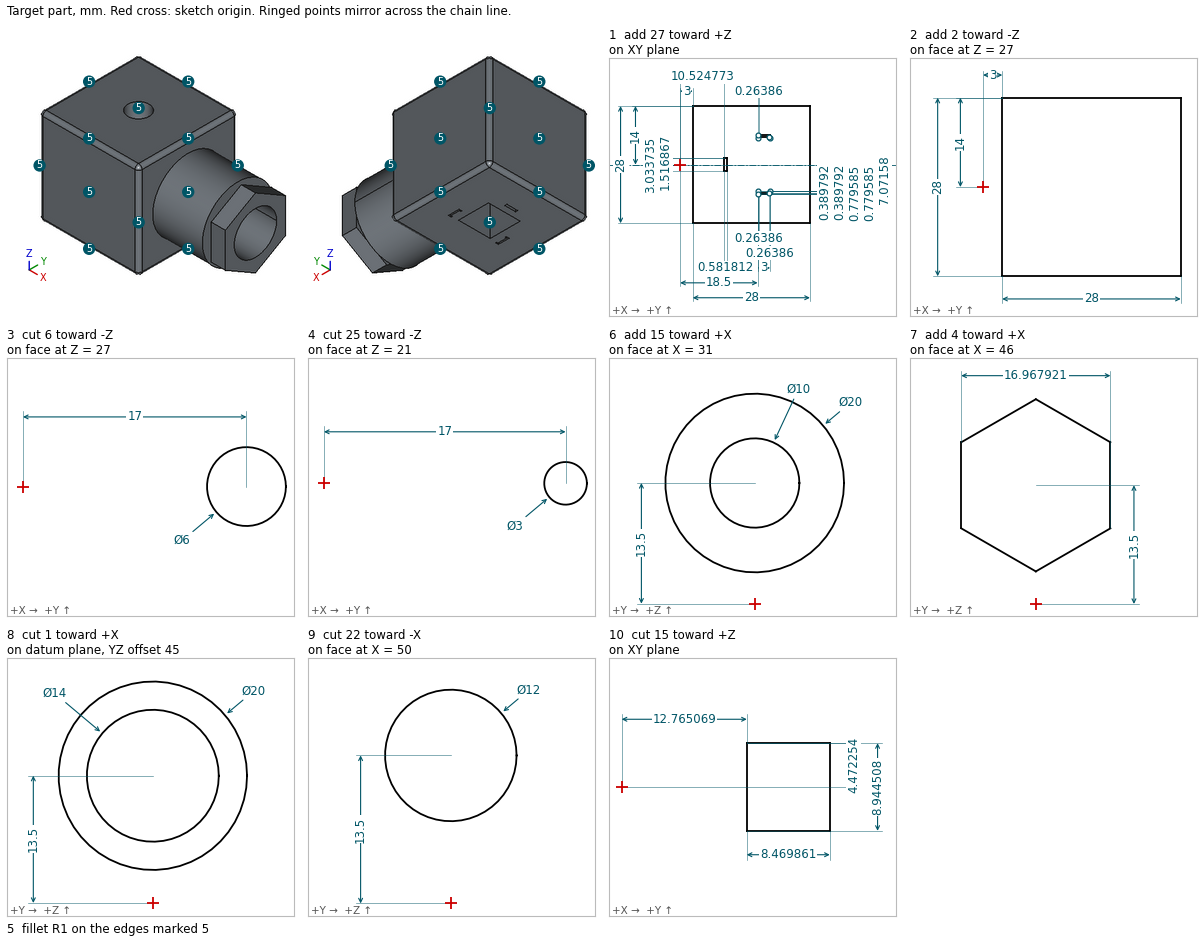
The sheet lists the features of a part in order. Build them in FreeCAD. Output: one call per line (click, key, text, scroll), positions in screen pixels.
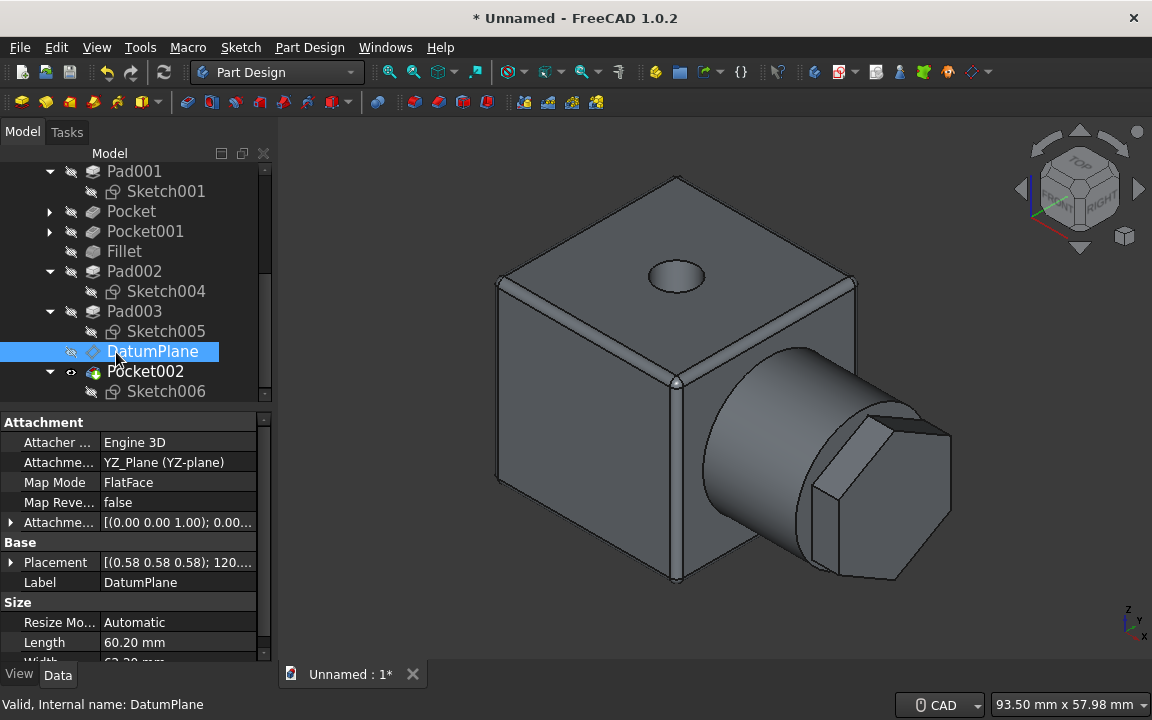
click(390, 72)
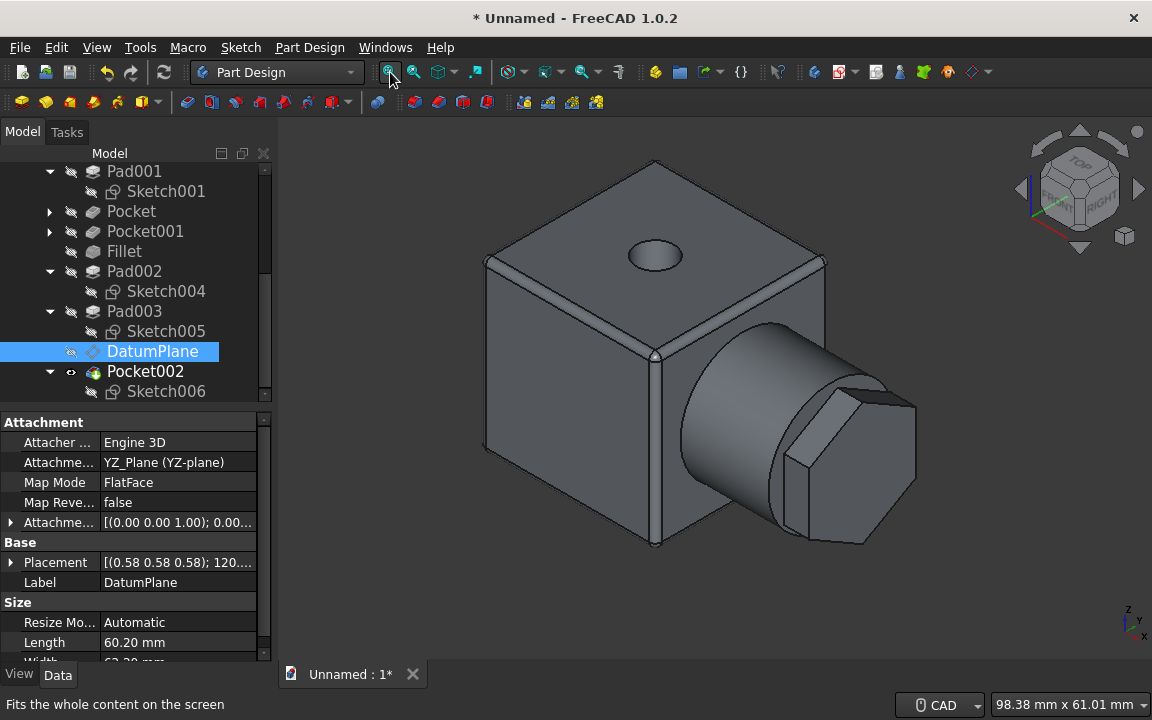
click(863, 472)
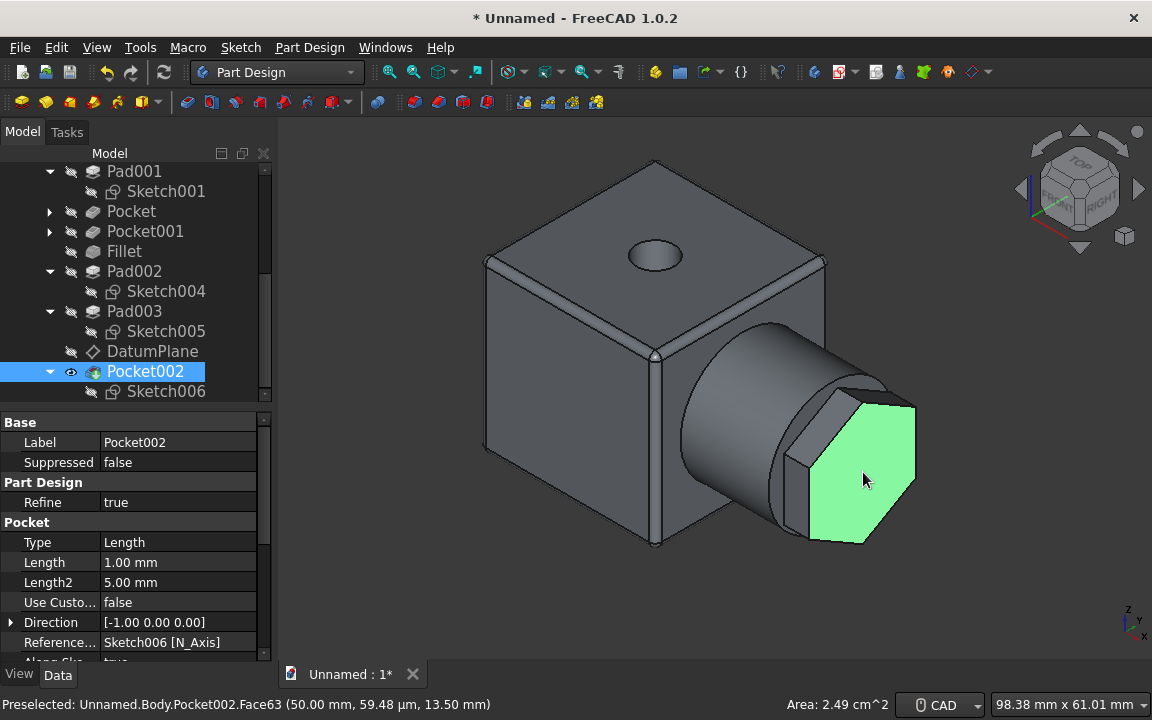
click(840, 72)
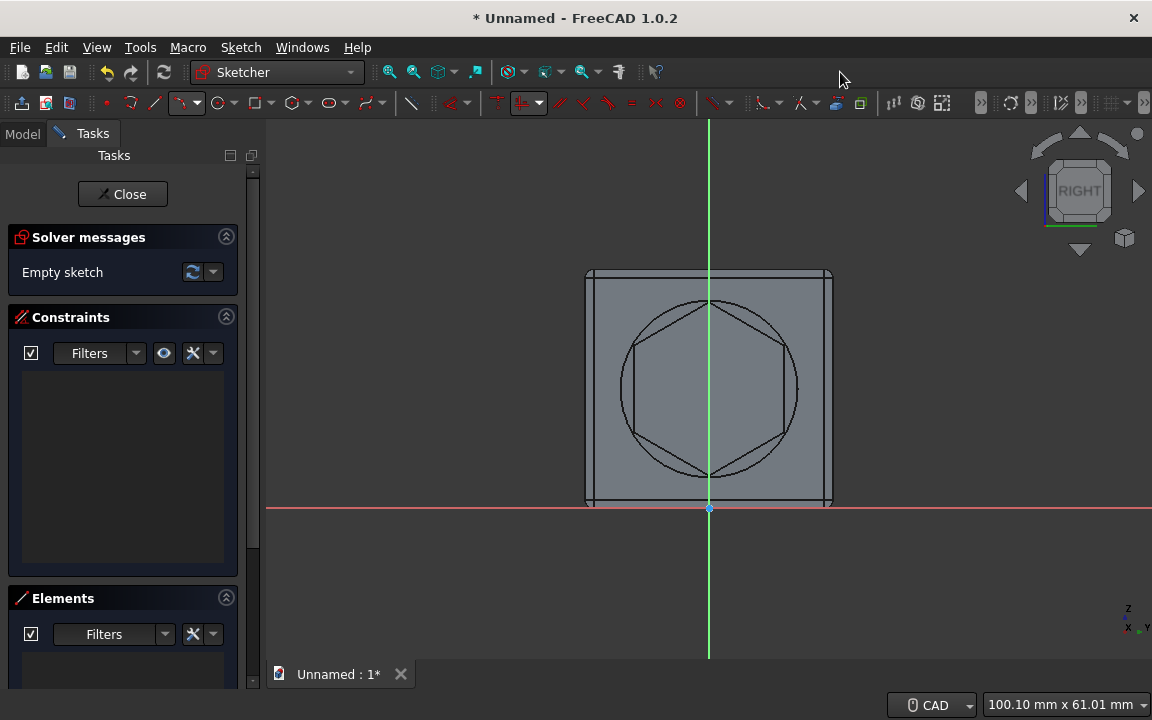
scroll(792, 463, up, 3)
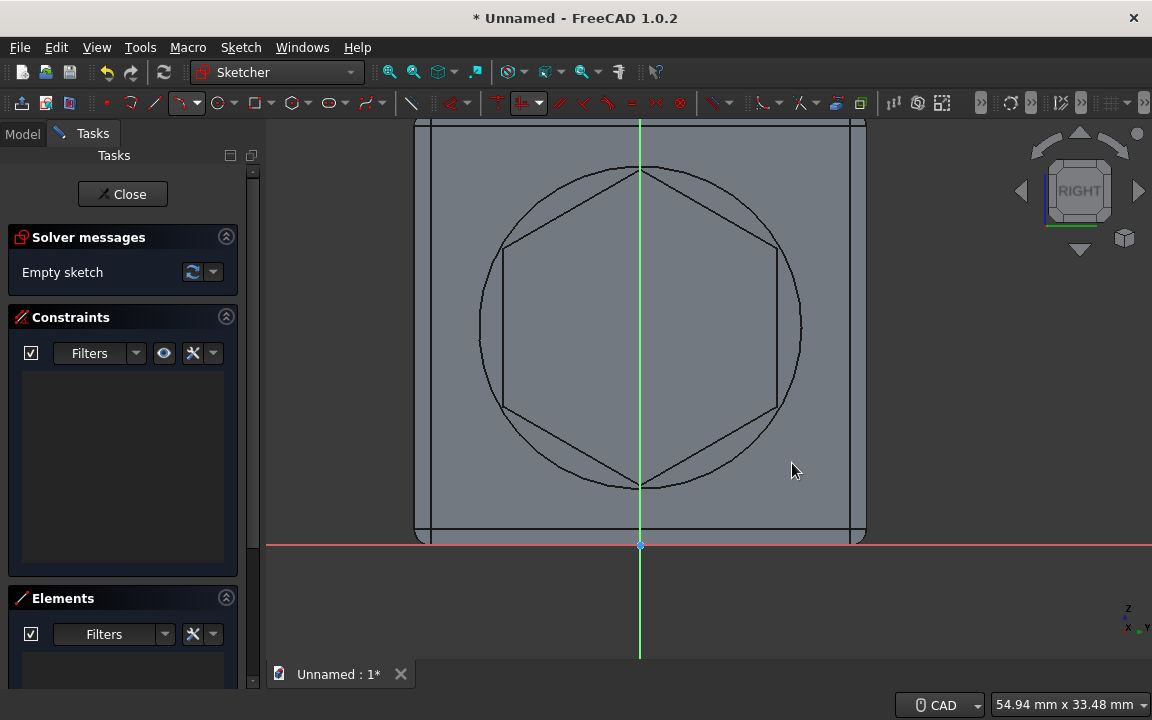
click(218, 104)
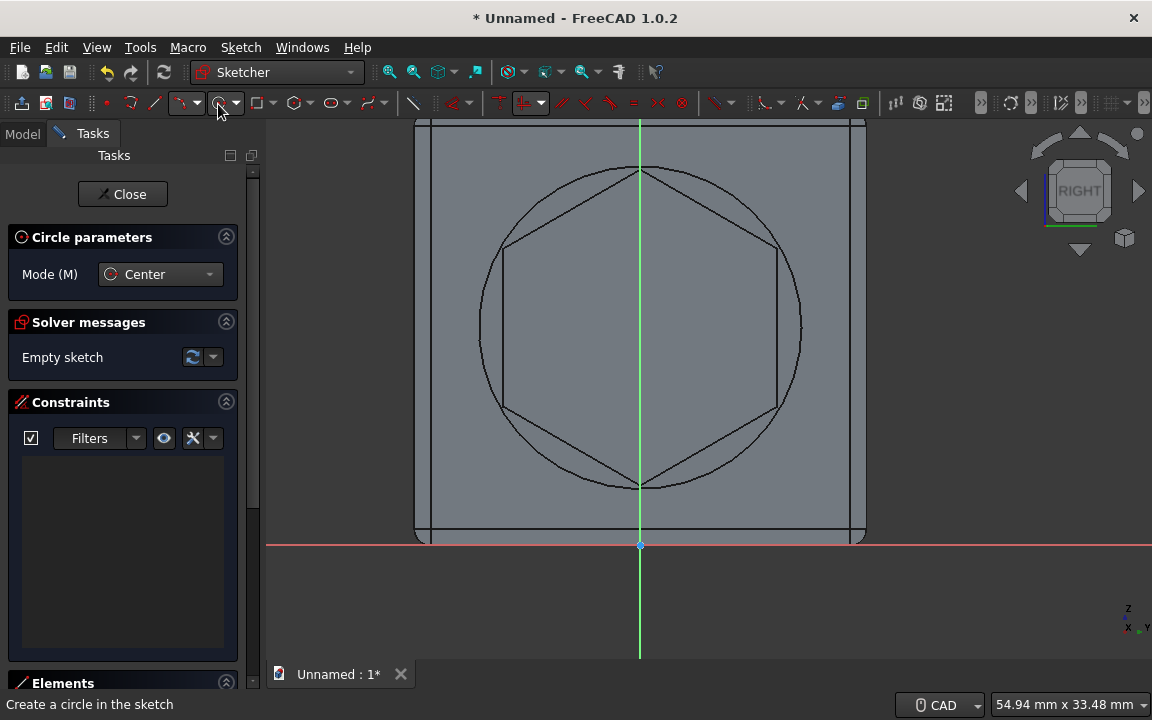
click(640, 328)
click(709, 259)
key(Escape)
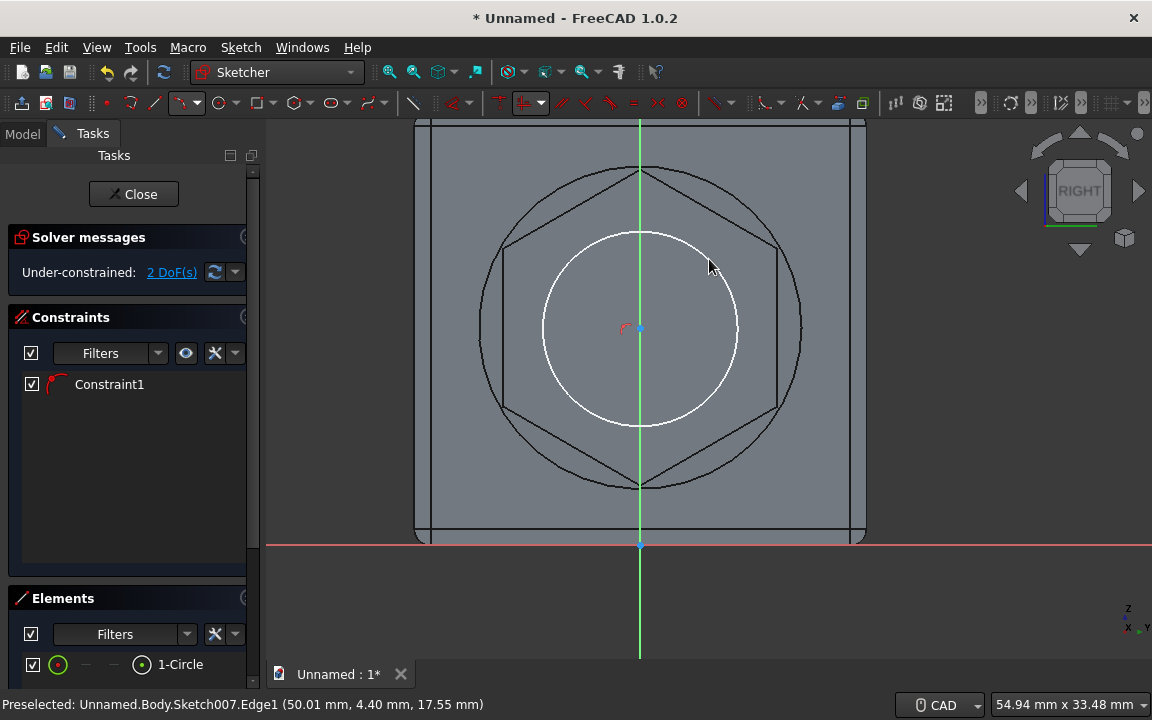
click(452, 104)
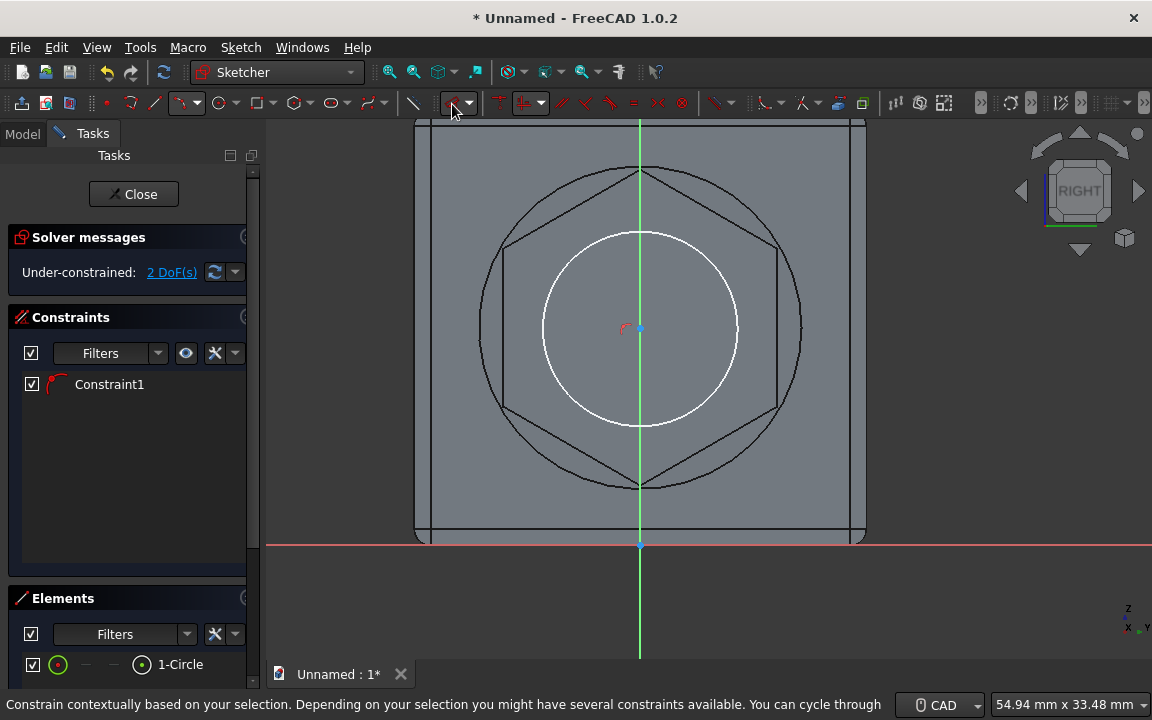
click(709, 260)
click(732, 237)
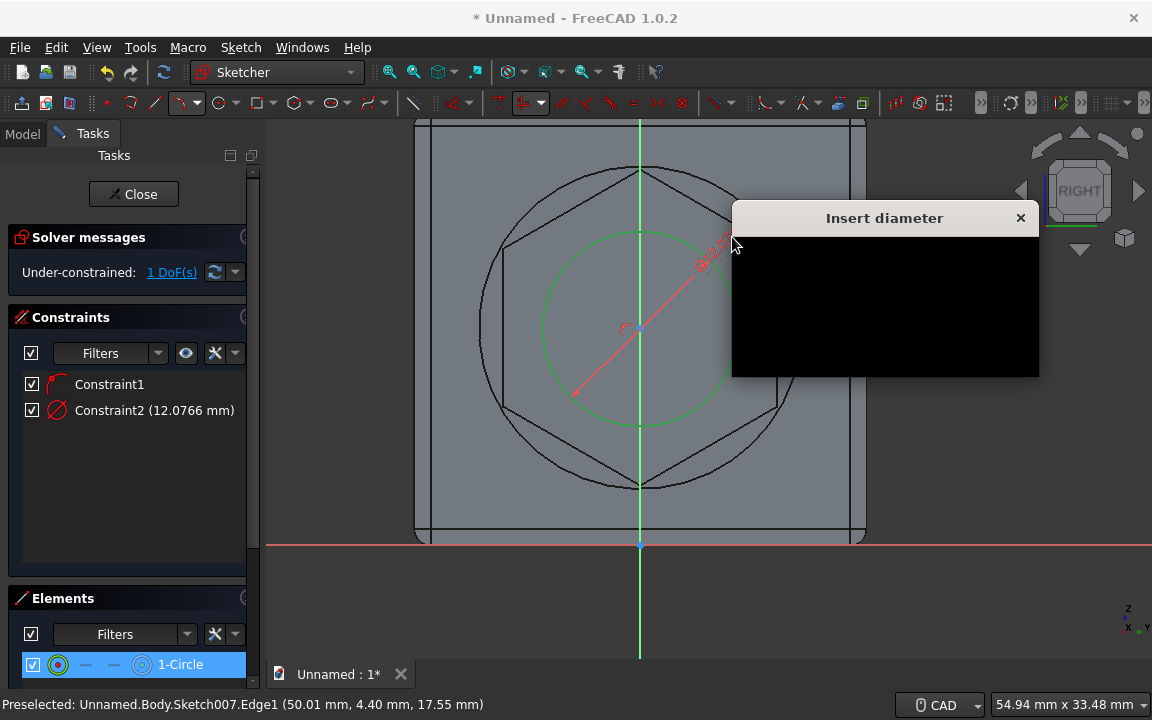
text(12)
key(Return)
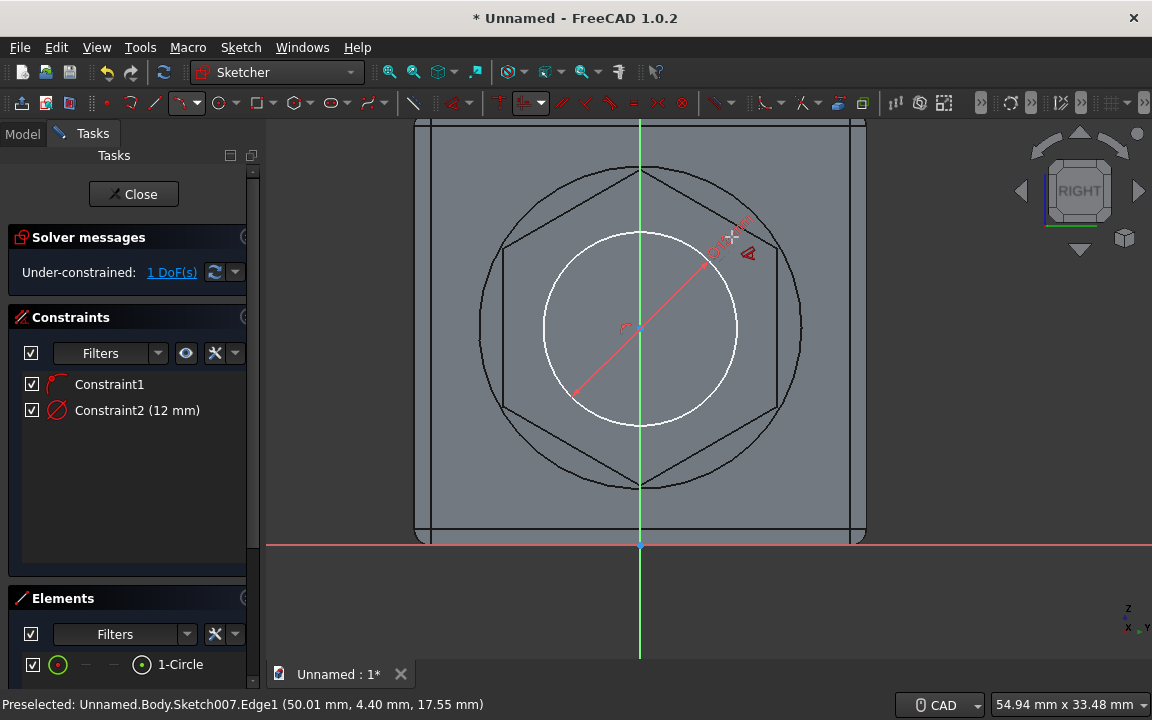
click(640, 329)
click(674, 437)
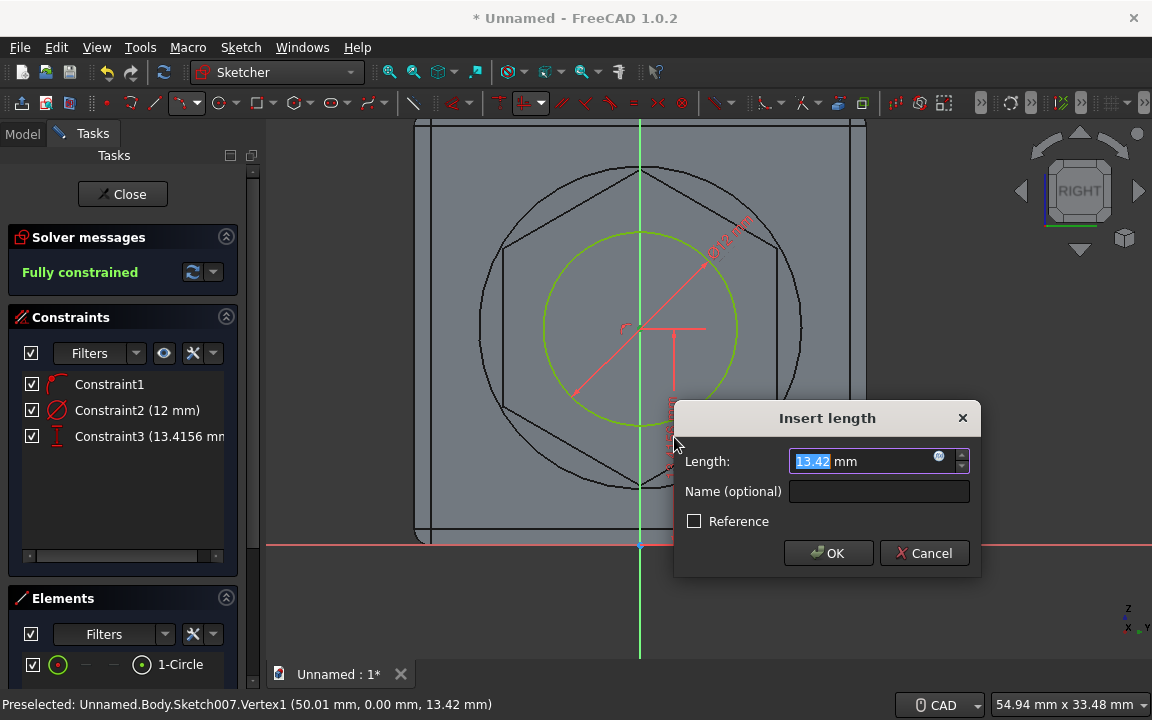
text(13.5)
key(Return)
key(Escape)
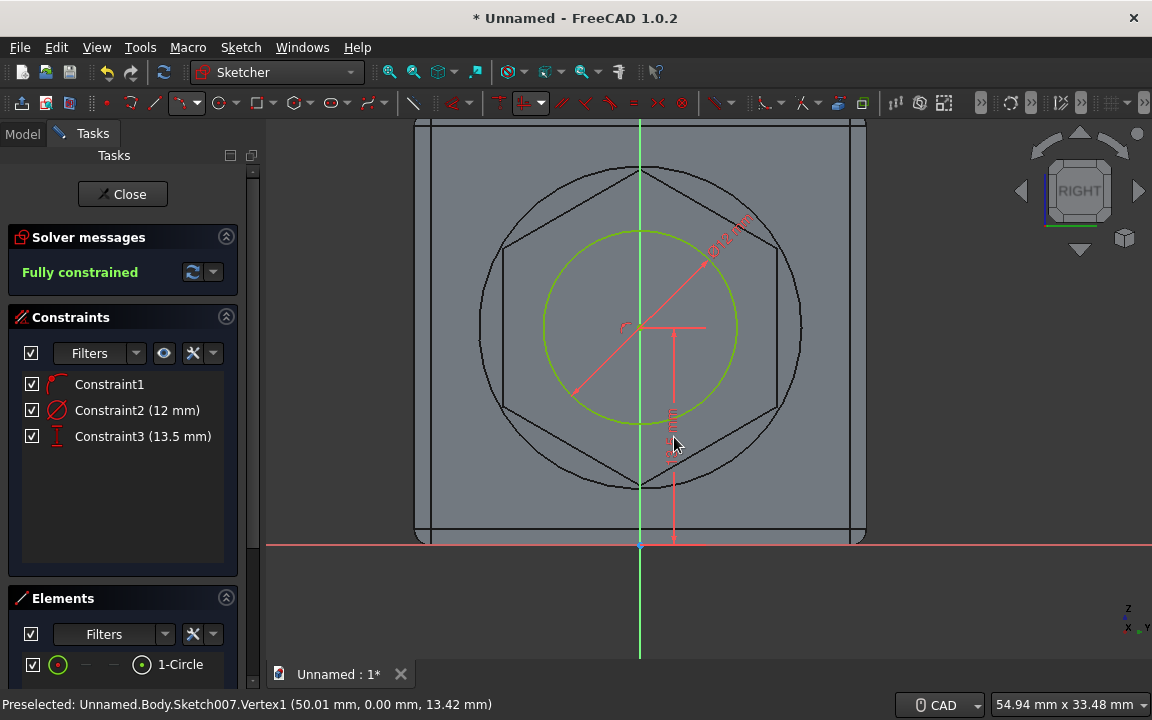
click(123, 194)